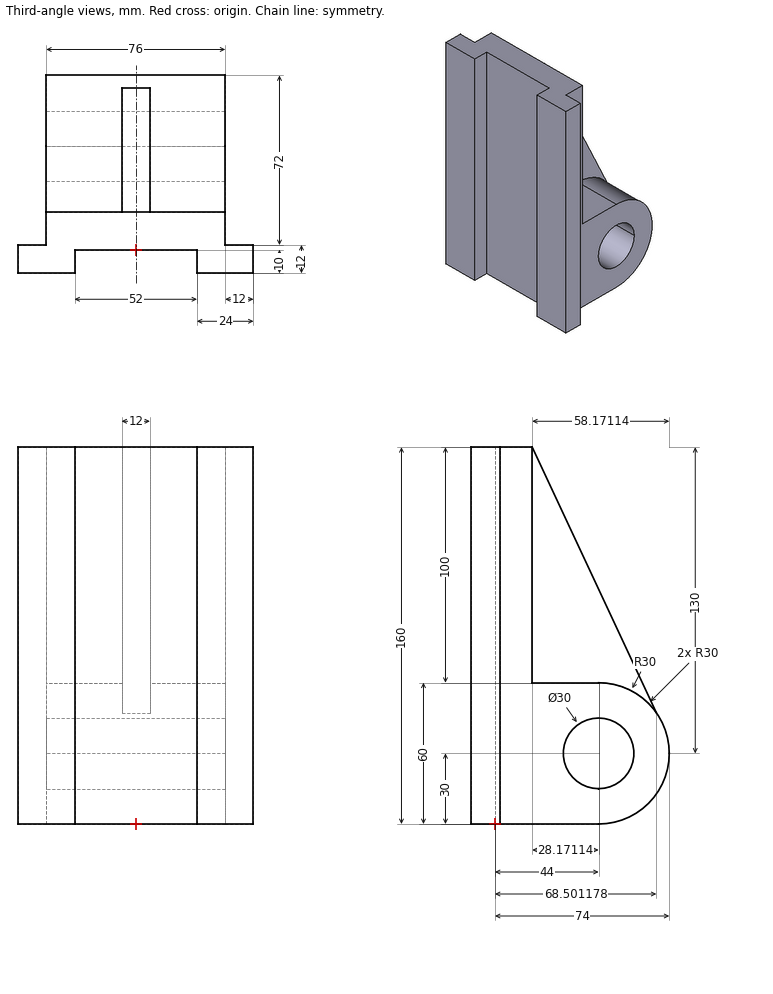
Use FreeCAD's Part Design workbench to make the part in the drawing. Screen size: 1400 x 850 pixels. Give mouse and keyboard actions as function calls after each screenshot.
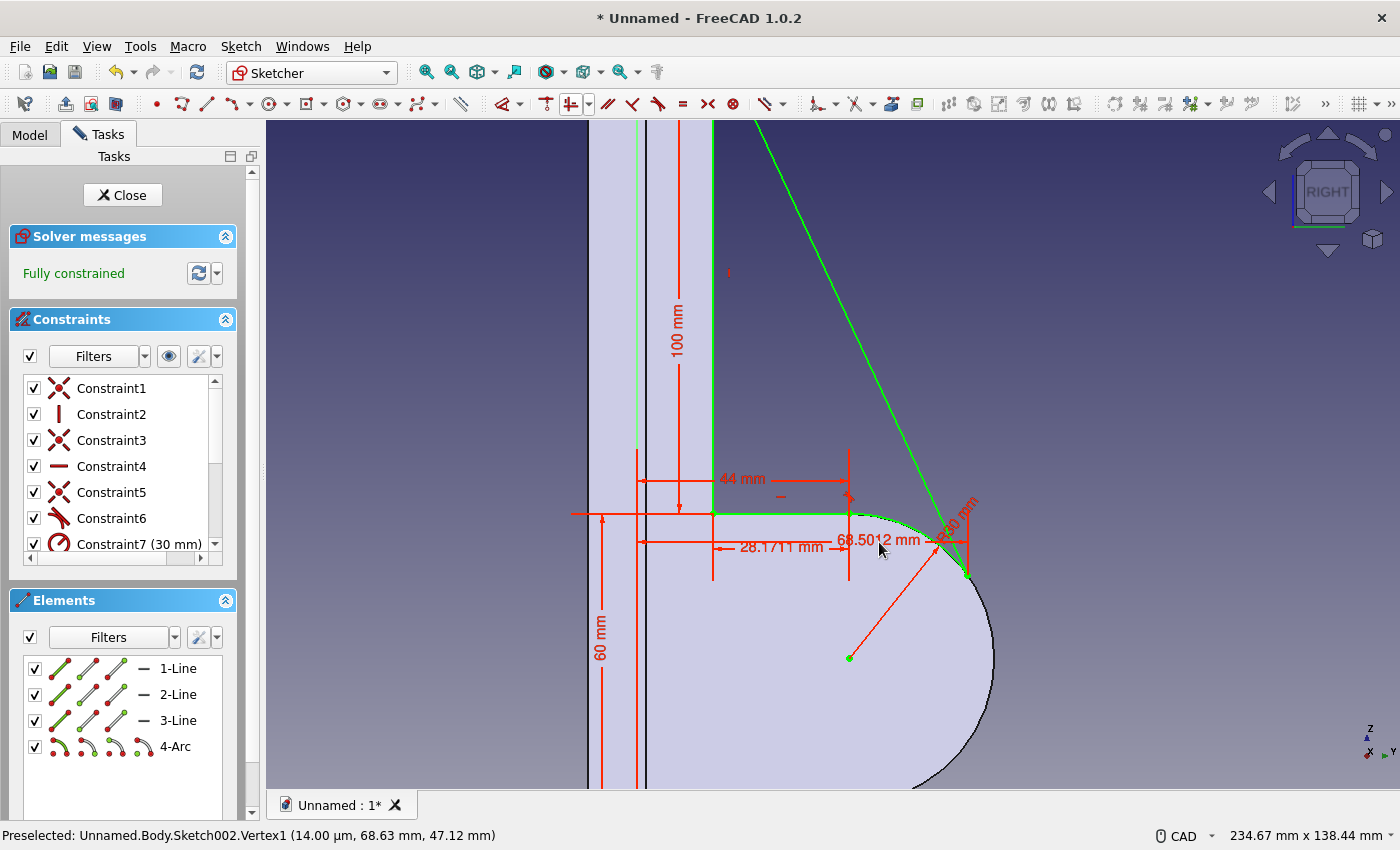
click(123, 195)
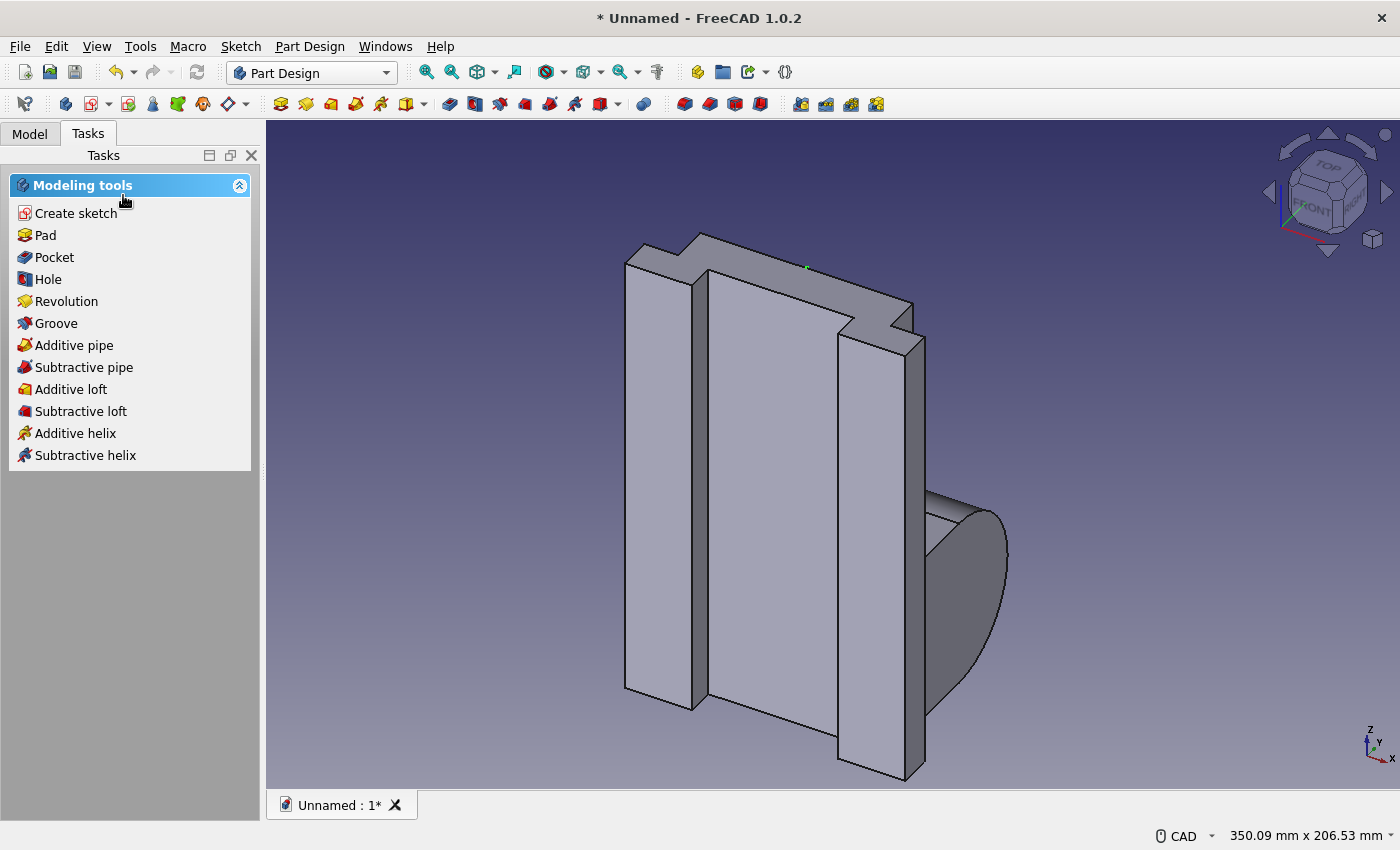
click(281, 104)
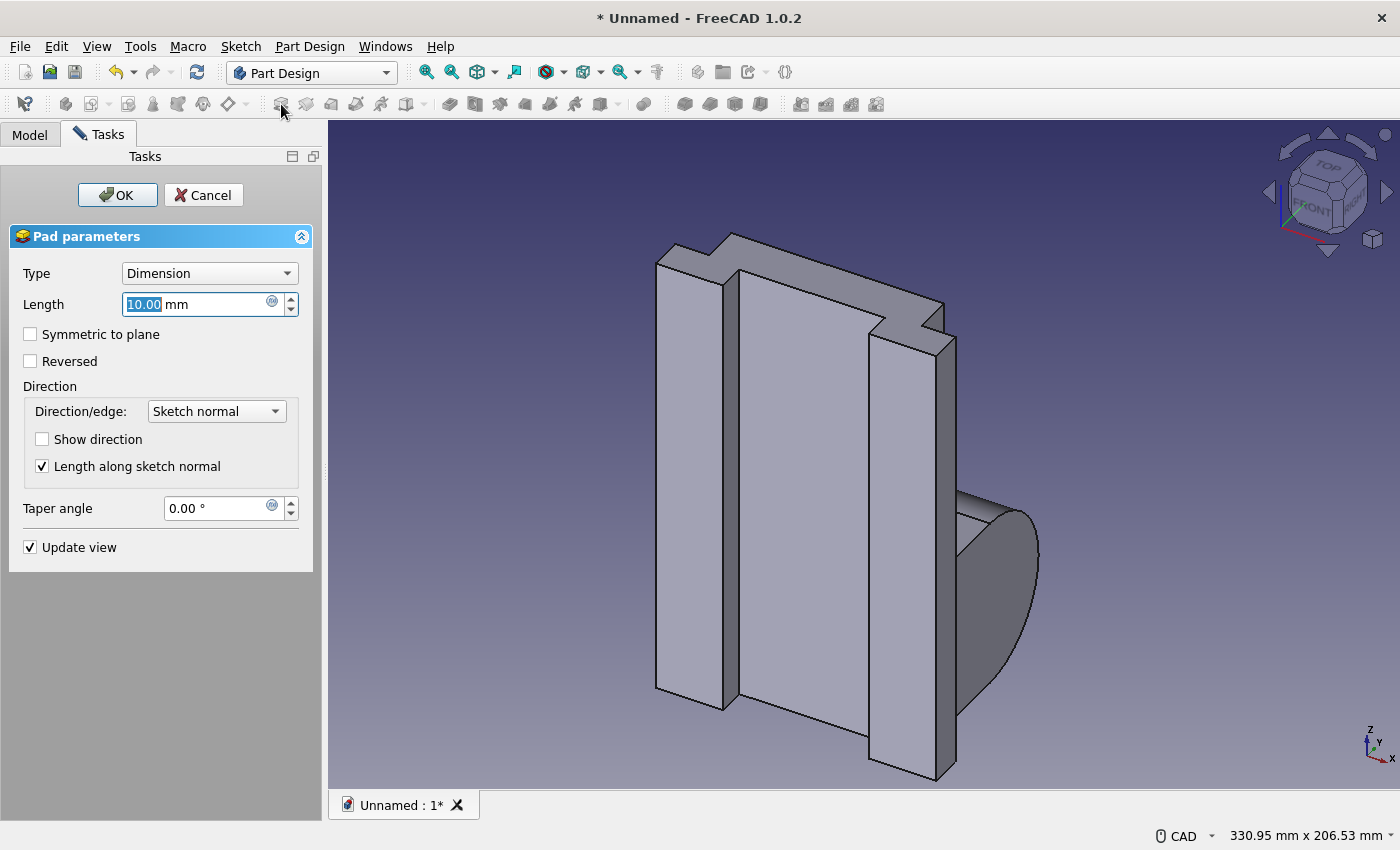
text(12)
key(Tab)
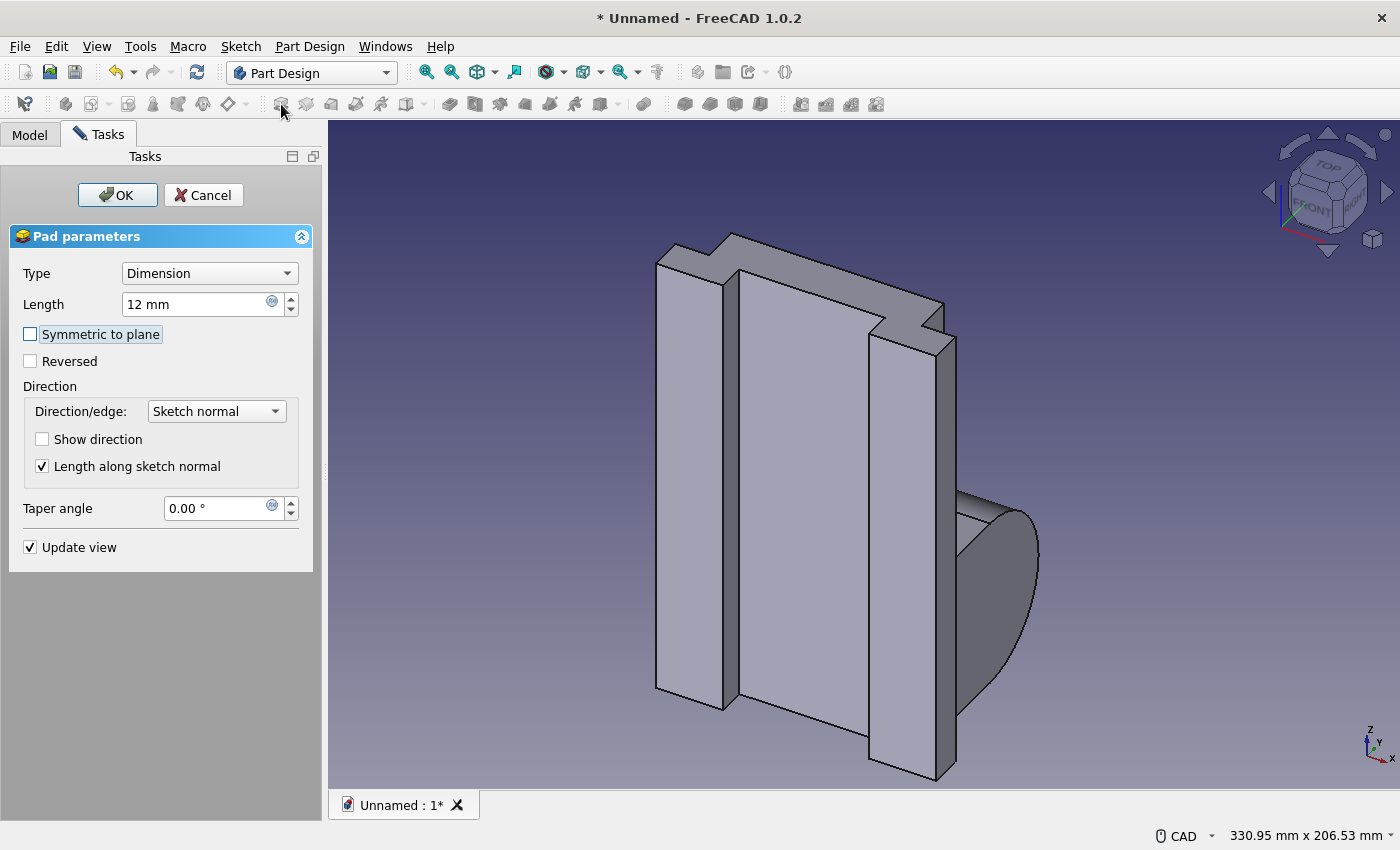
click(31, 334)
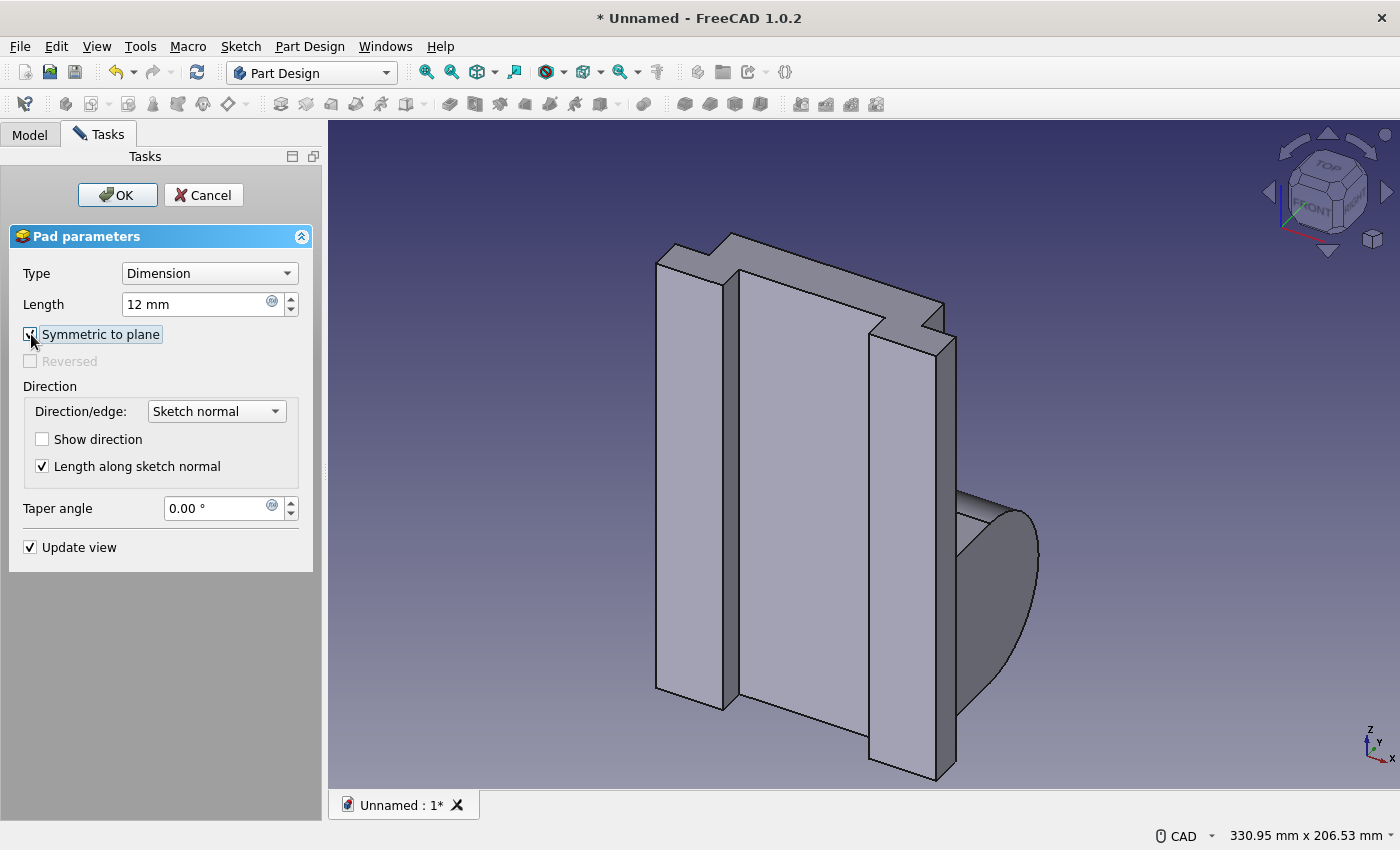
click(118, 195)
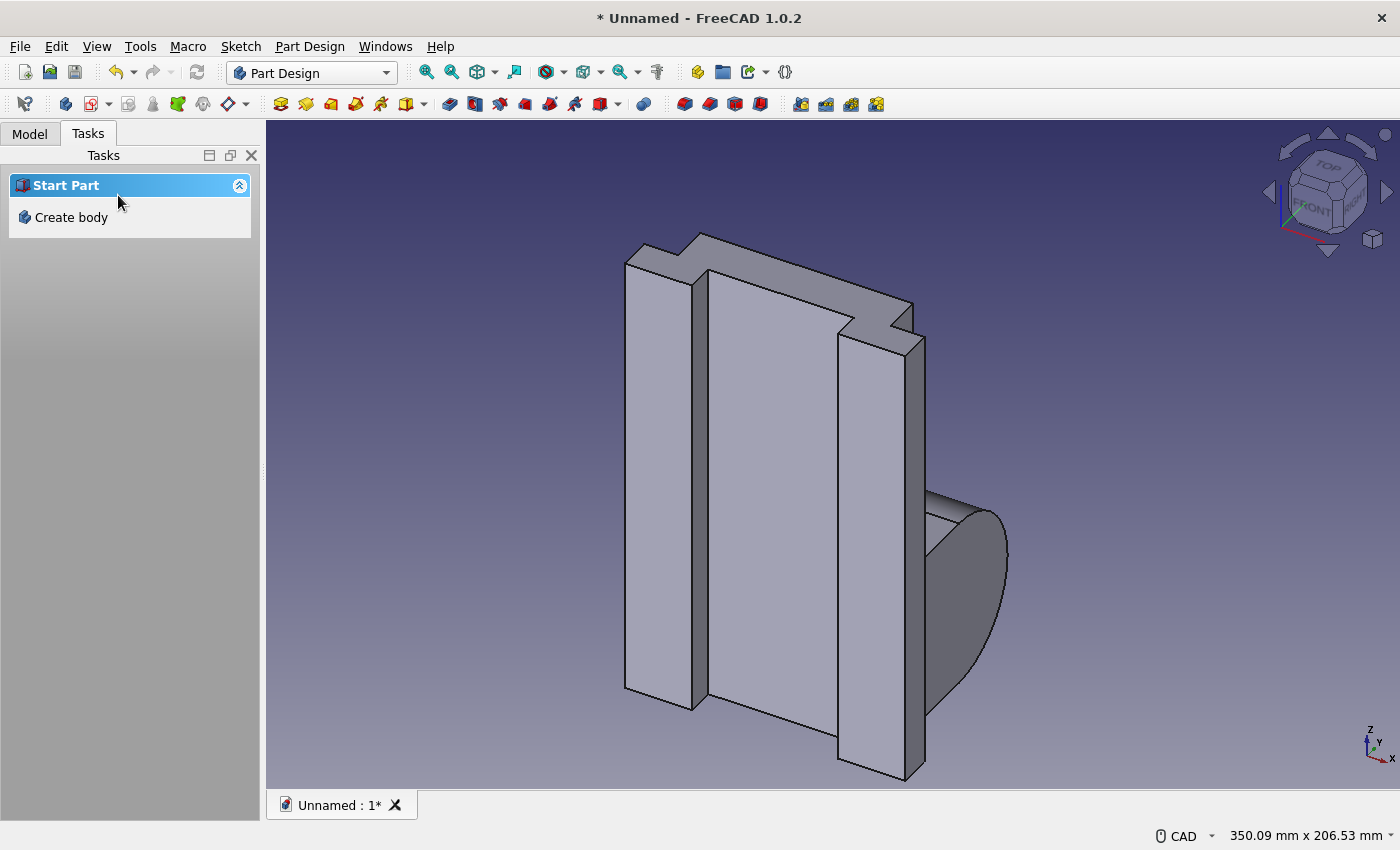
click(949, 600)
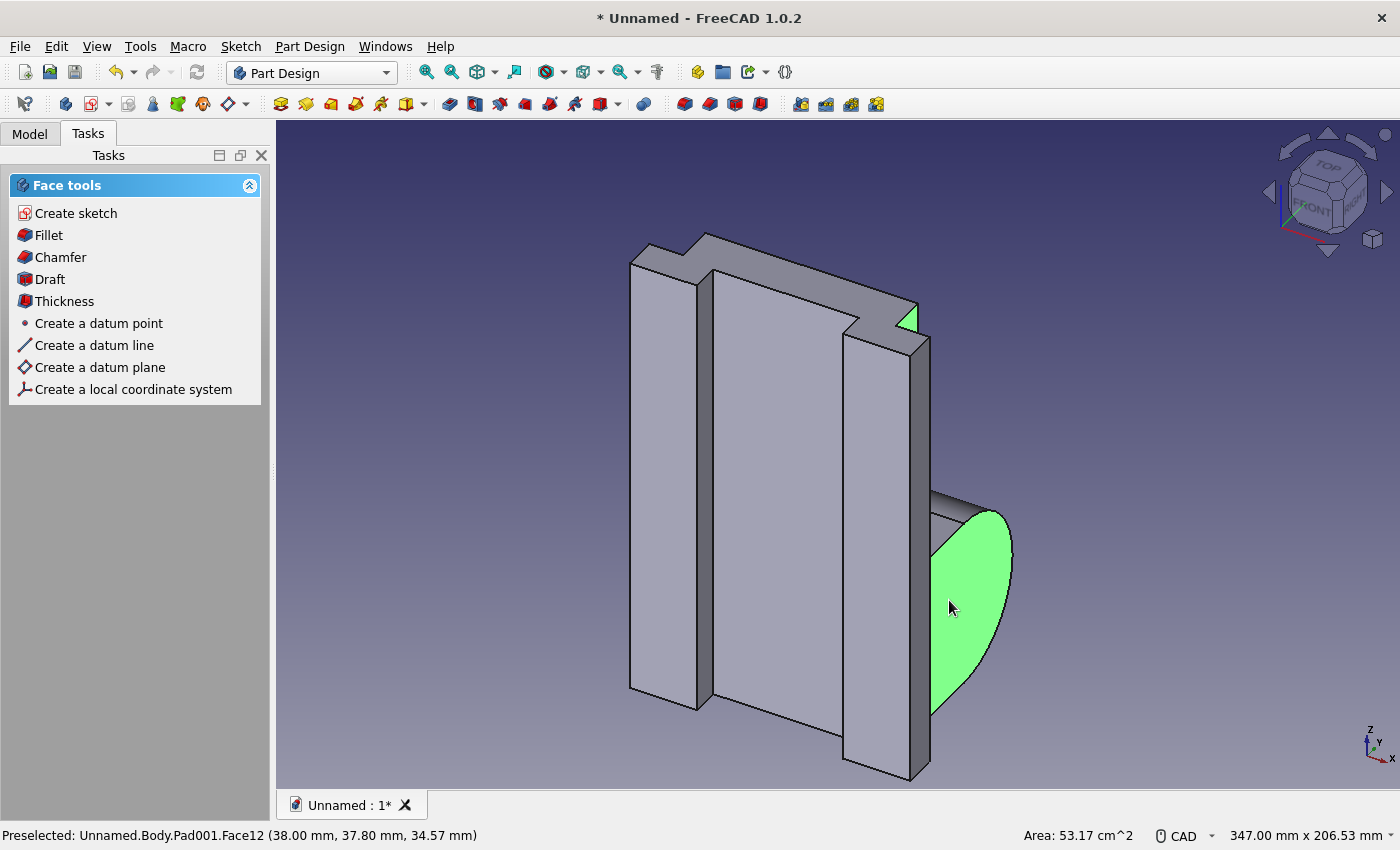
click(90, 104)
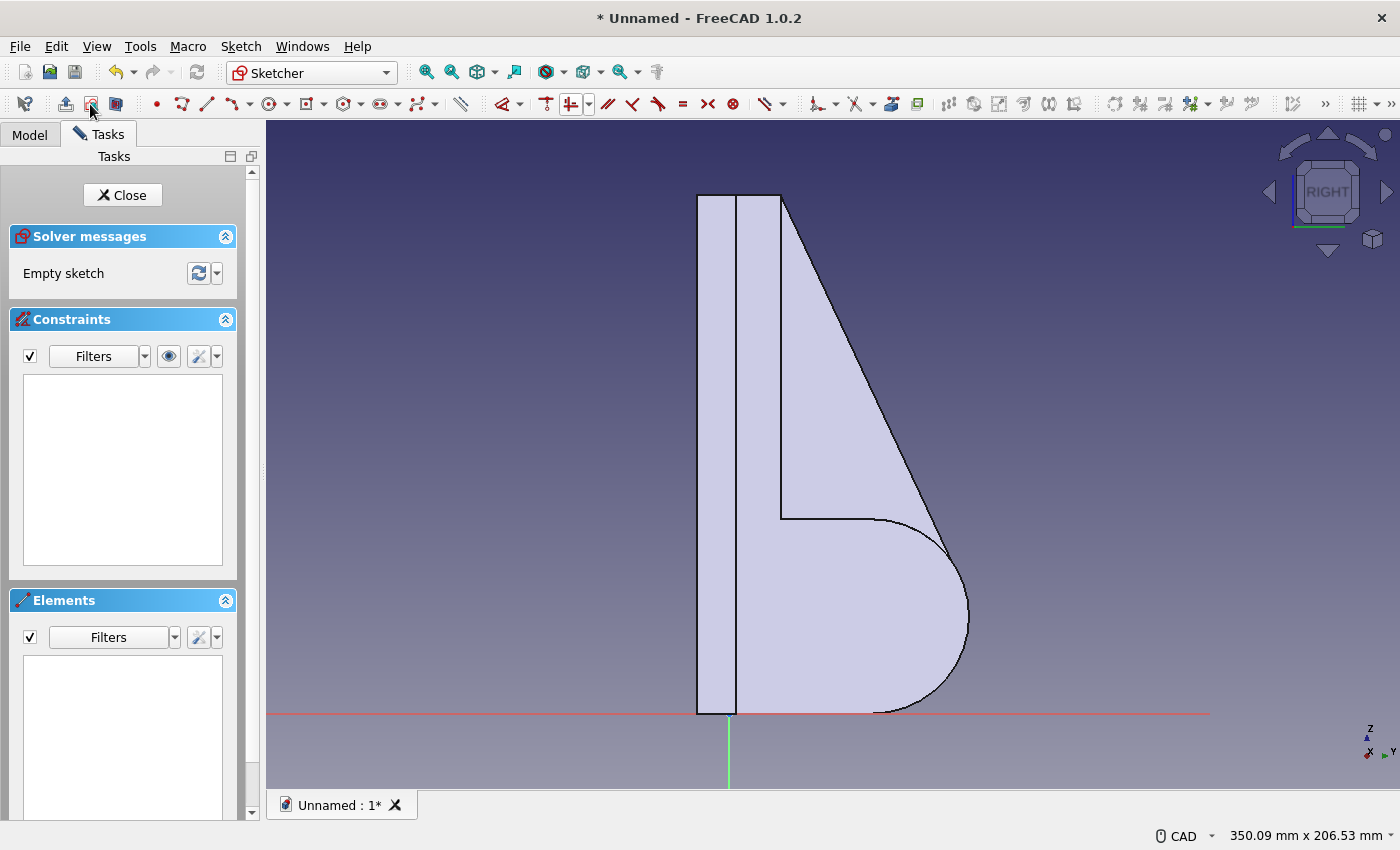
click(116, 104)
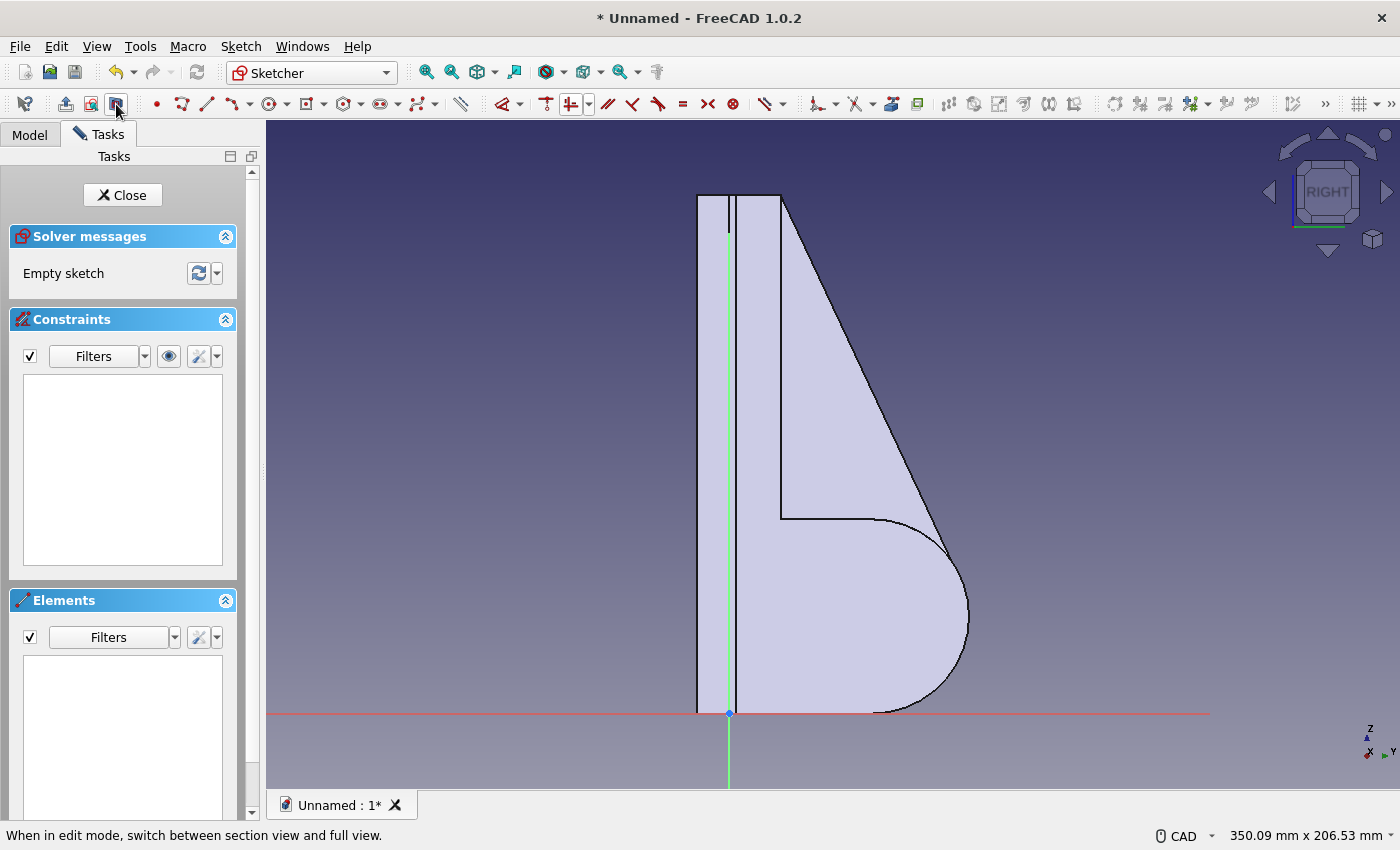
scroll(860, 749, up, 5)